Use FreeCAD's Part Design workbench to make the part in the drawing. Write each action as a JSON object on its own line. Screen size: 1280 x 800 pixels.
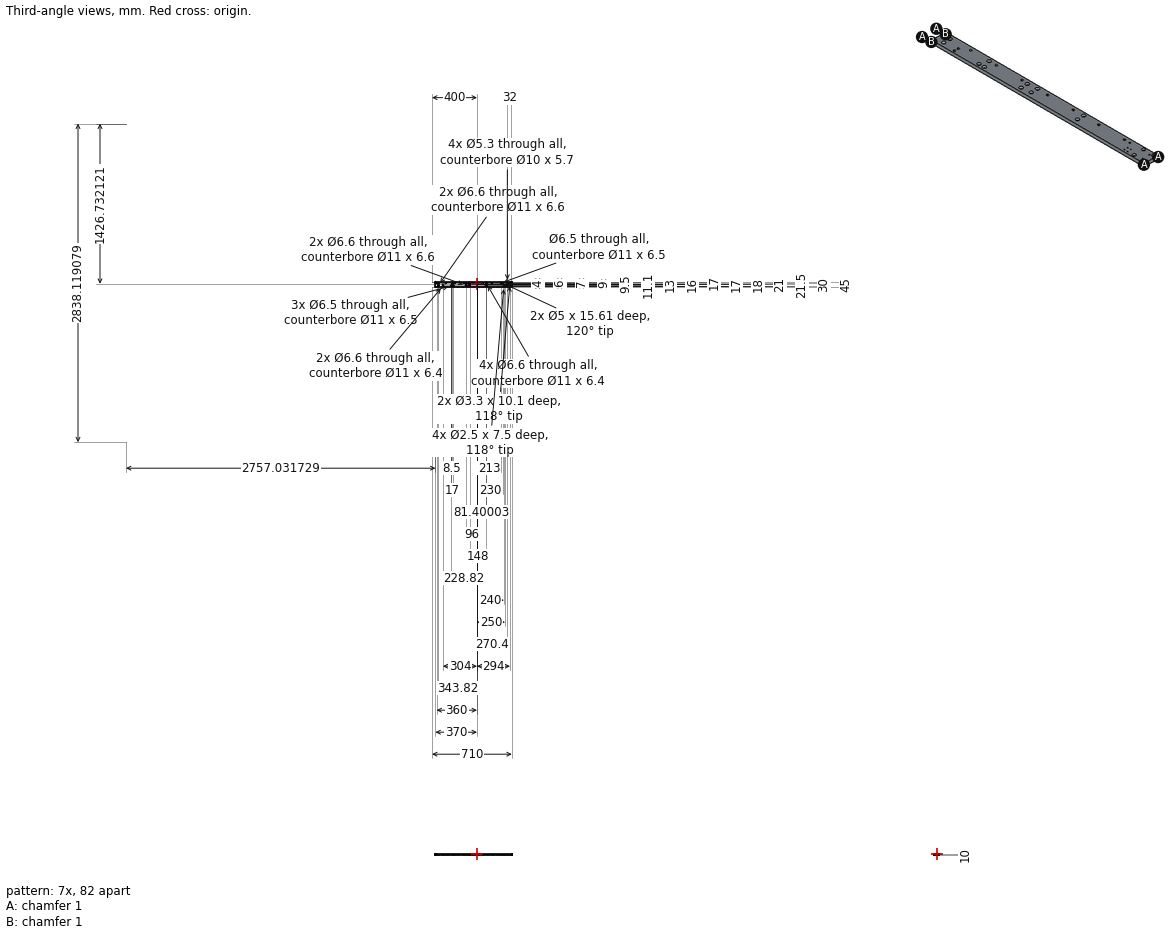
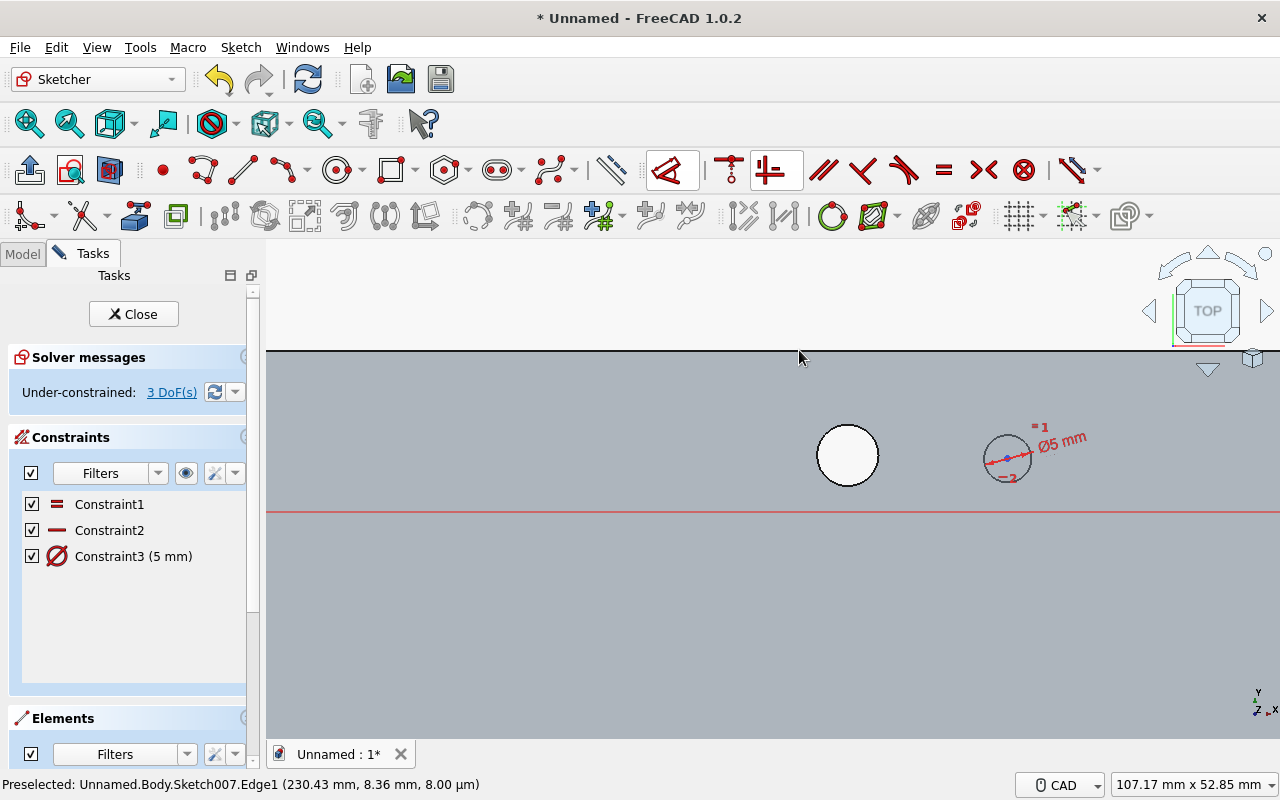
{"action": "left_click", "coordinate": [1008, 459]}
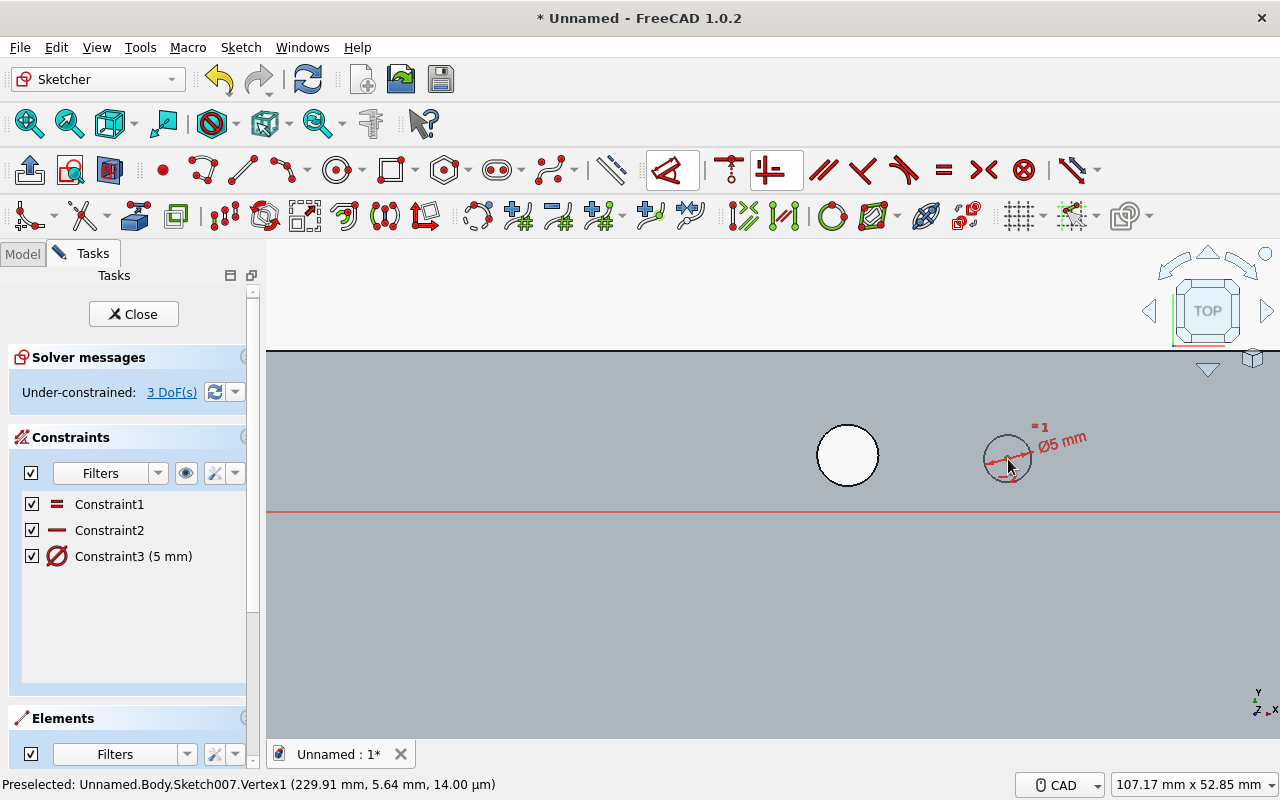
{"action": "left_click", "coordinate": [694, 170]}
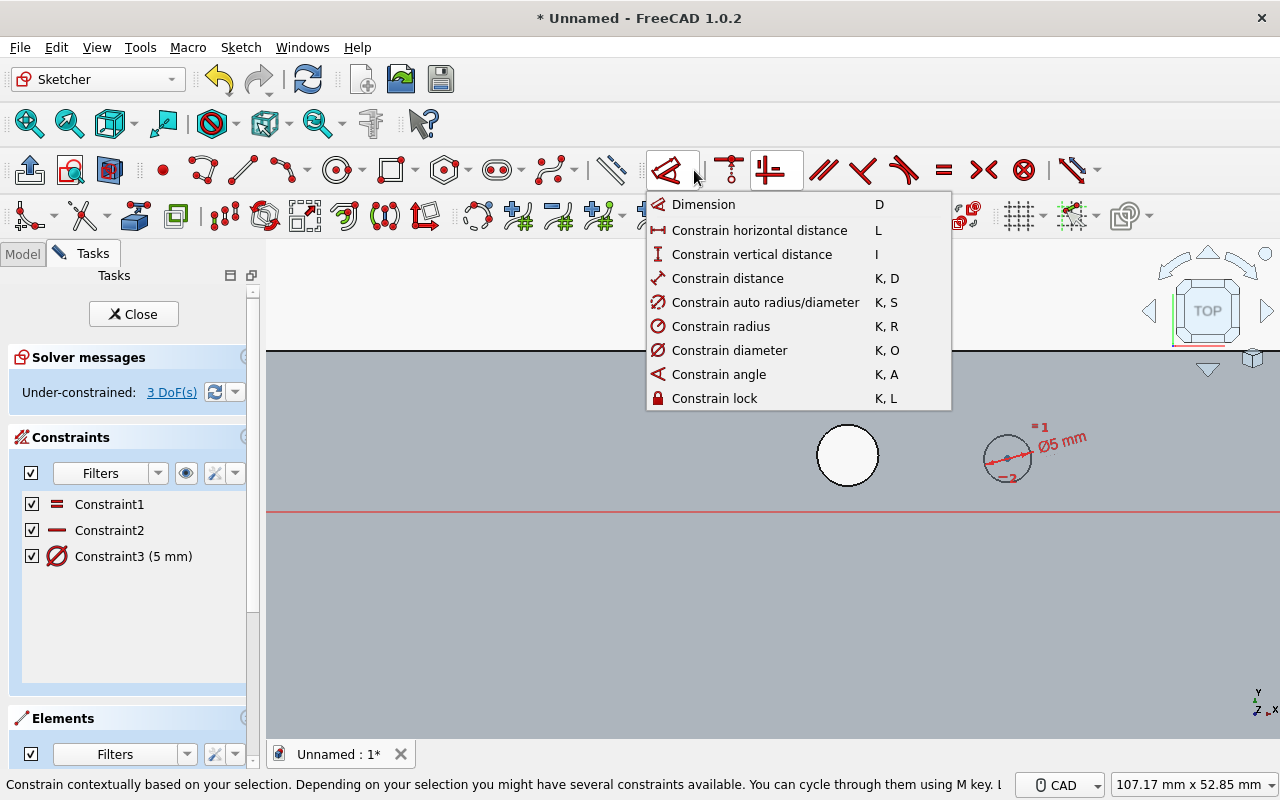
{"action": "left_click", "coordinate": [799, 254]}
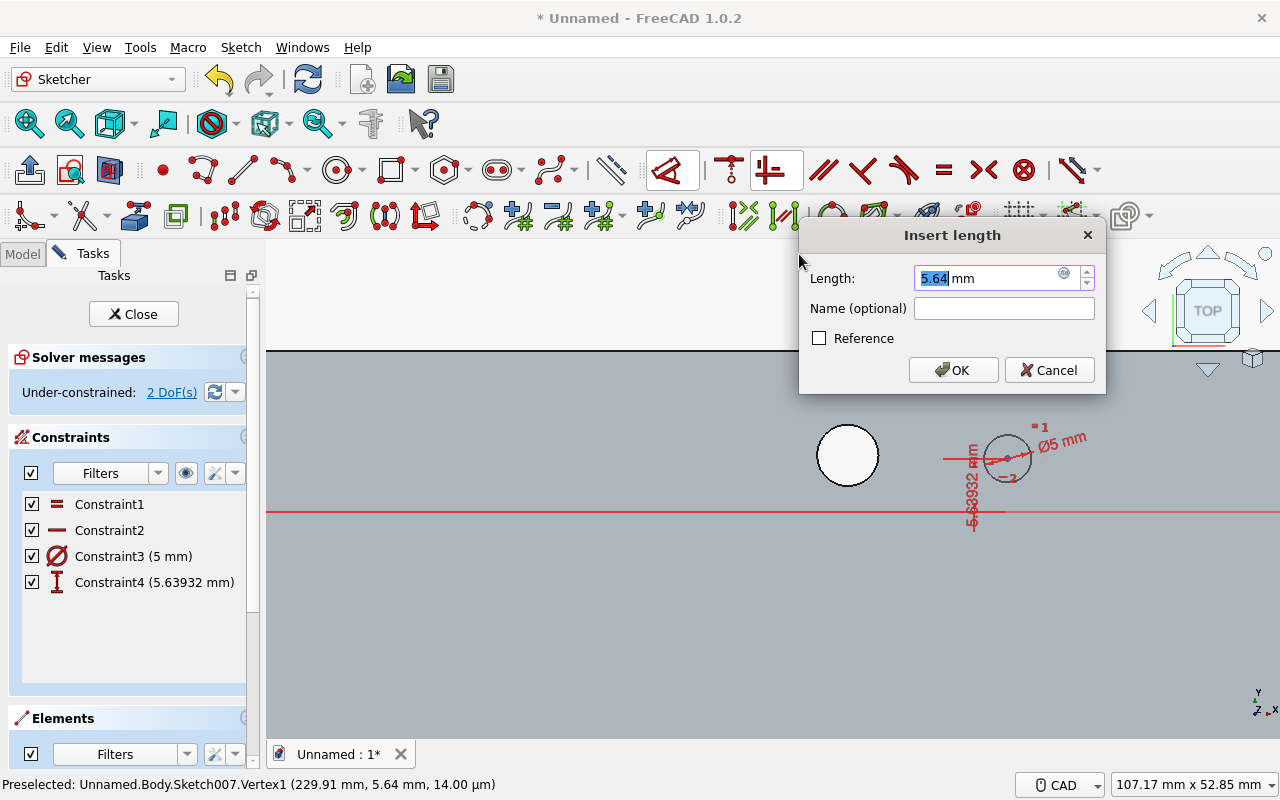
{"action": "type", "text": "6"}
{"action": "key", "text": "Return"}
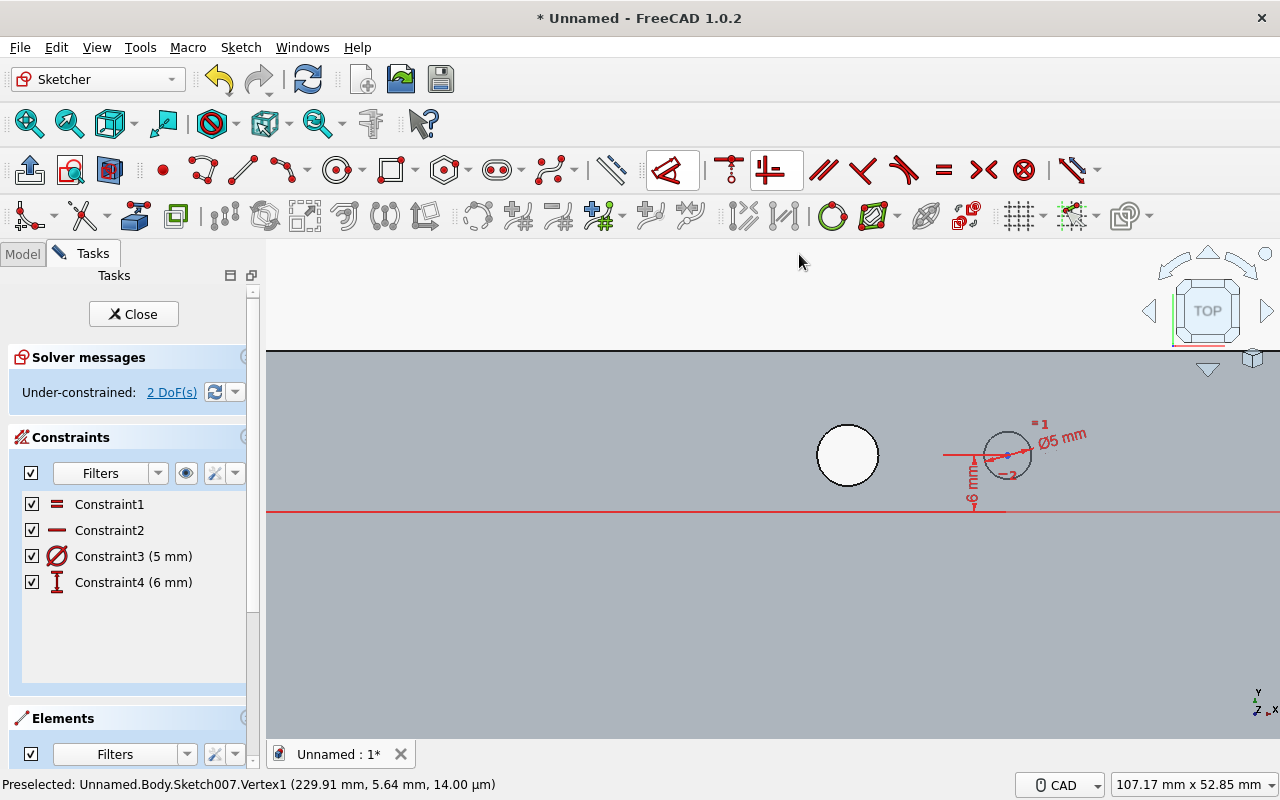
{"action": "scroll", "coordinate": [1014, 491], "scroll_direction": "down", "scroll_amount": 11}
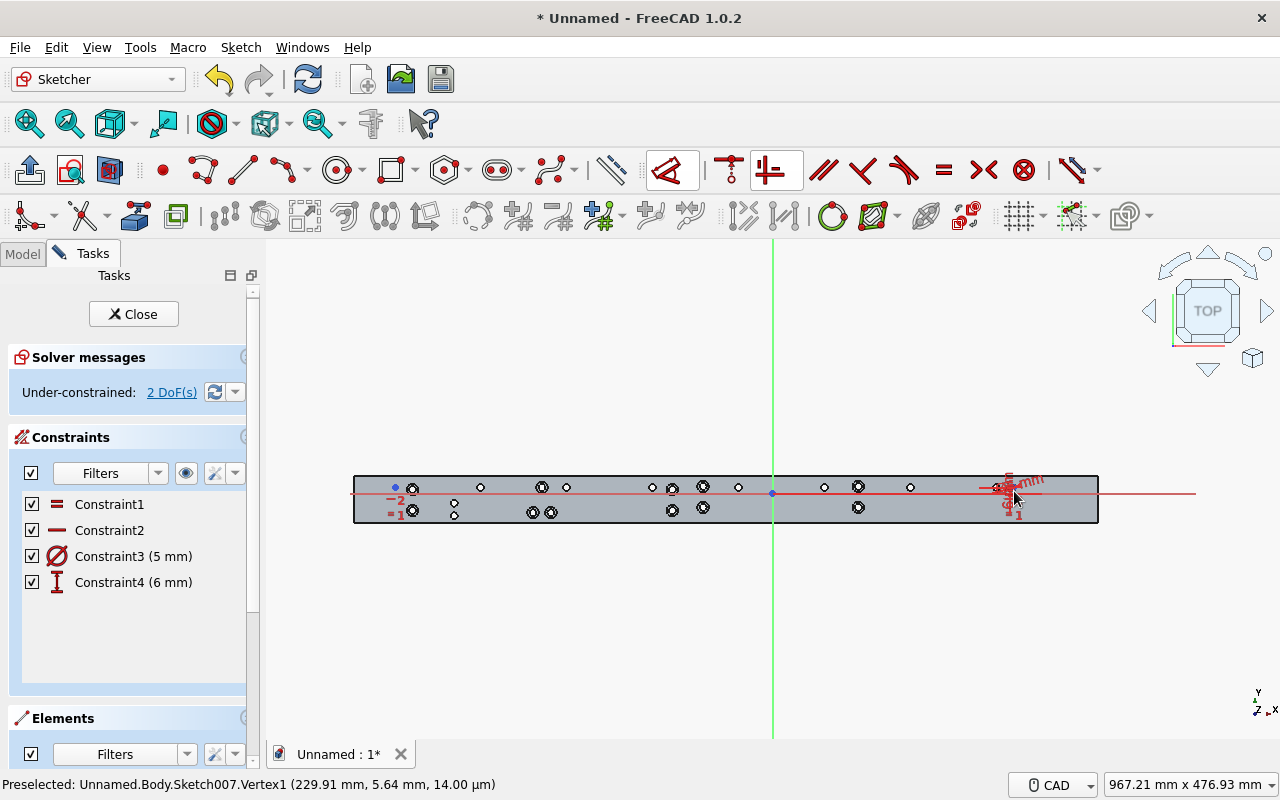
{"action": "left_click", "coordinate": [1014, 488]}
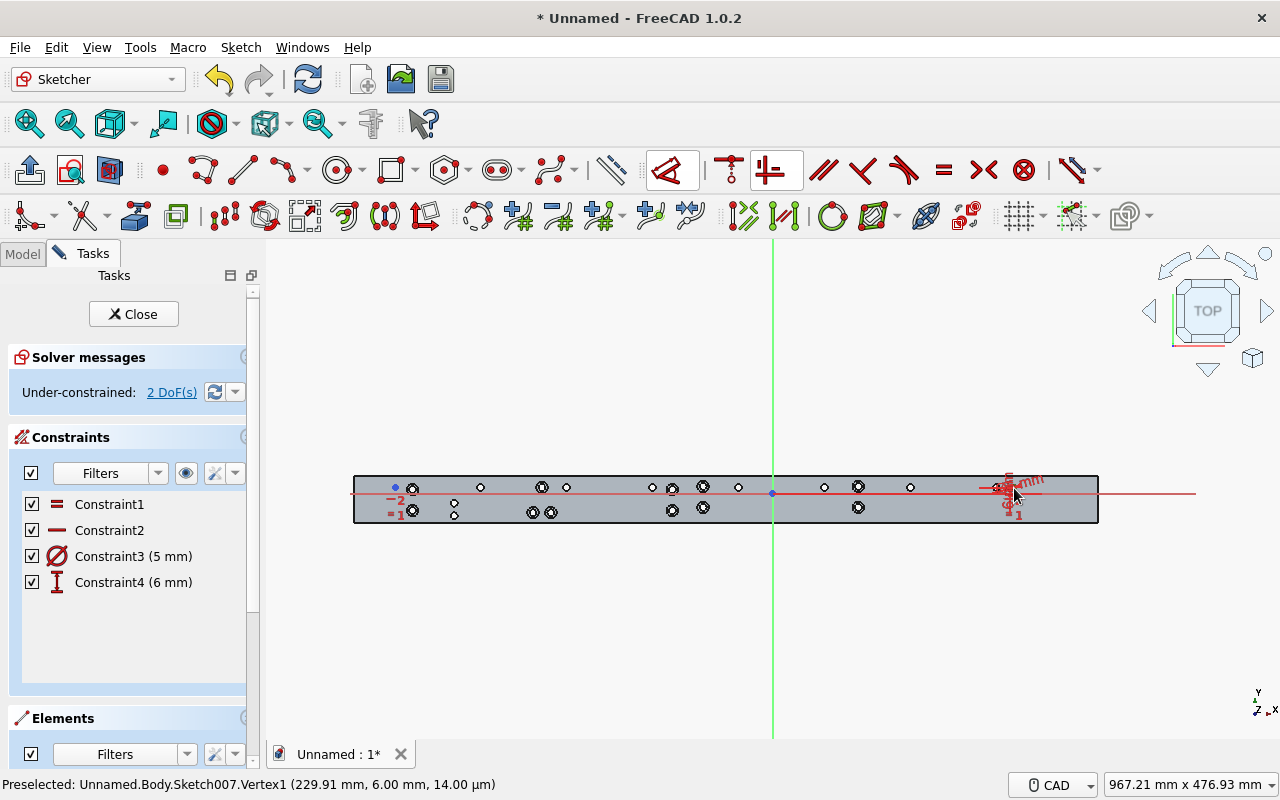
{"action": "key", "text": "l"}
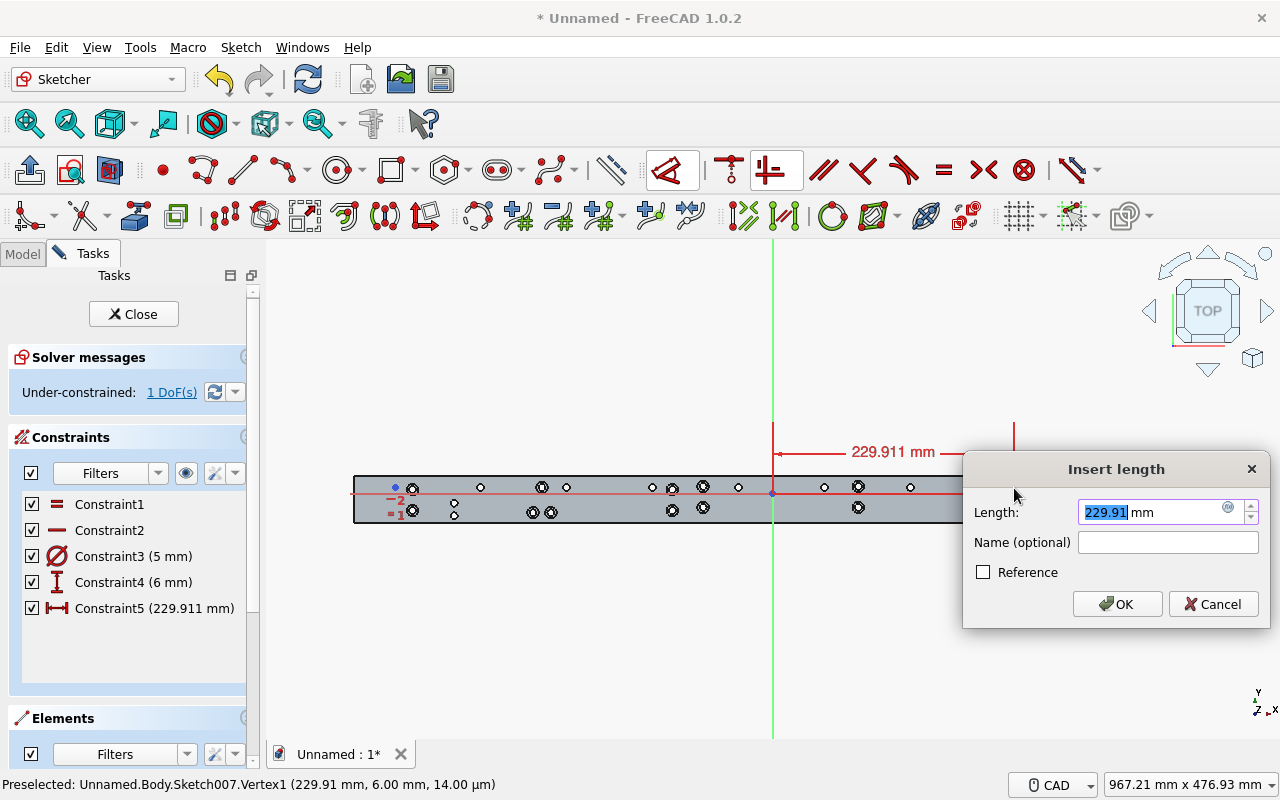
{"action": "type", "text": "230"}
{"action": "key", "text": "Return"}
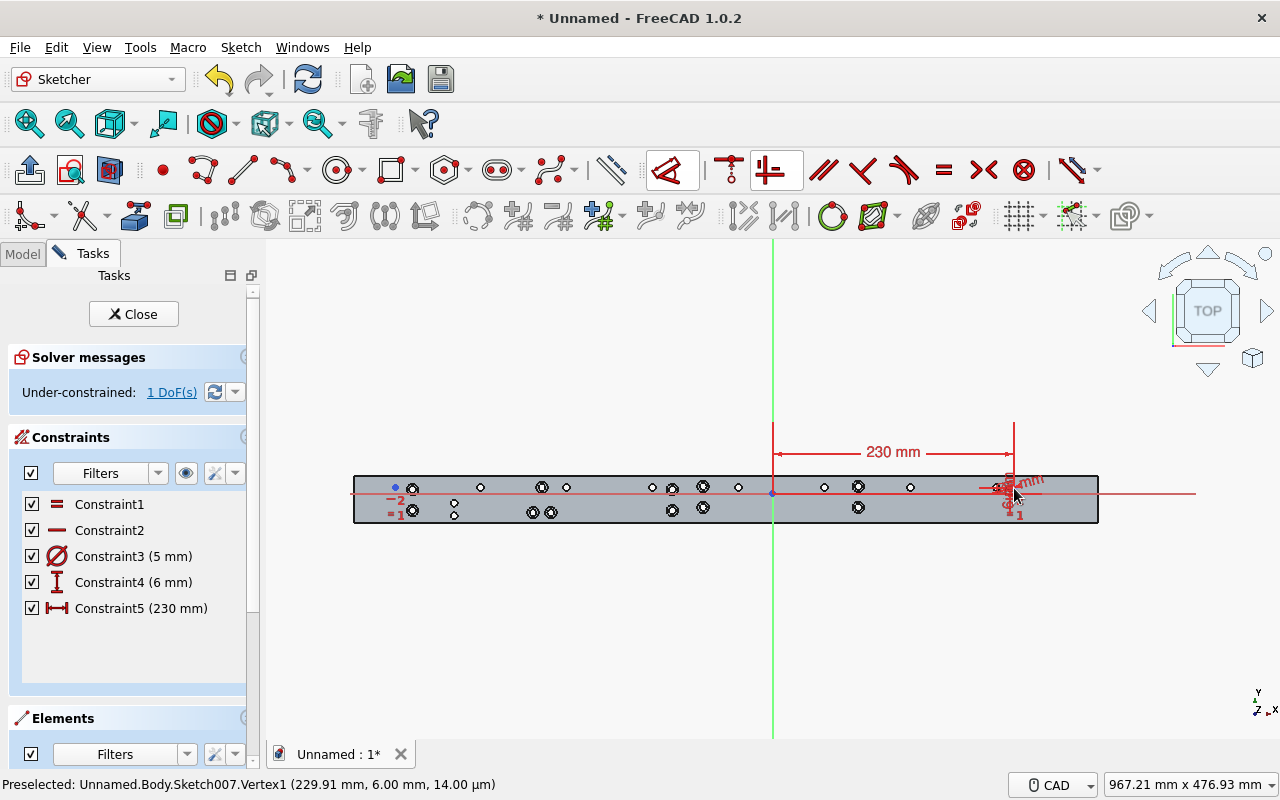
{"action": "left_click", "coordinate": [396, 488]}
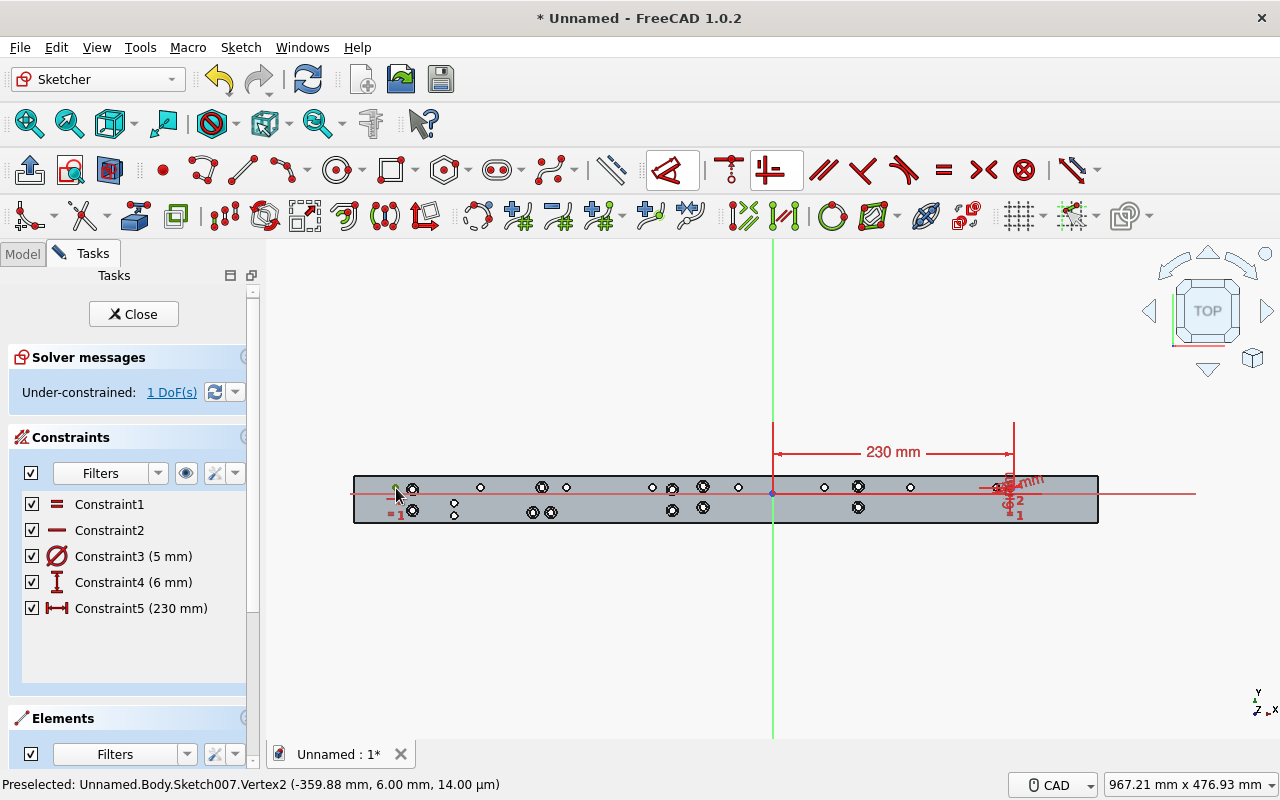
{"action": "key", "text": "l"}